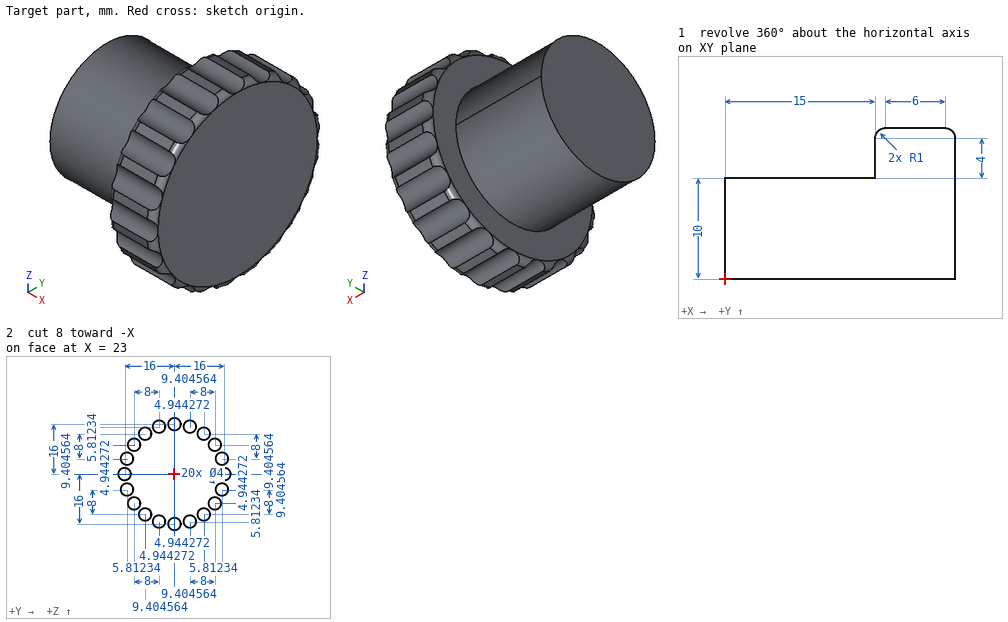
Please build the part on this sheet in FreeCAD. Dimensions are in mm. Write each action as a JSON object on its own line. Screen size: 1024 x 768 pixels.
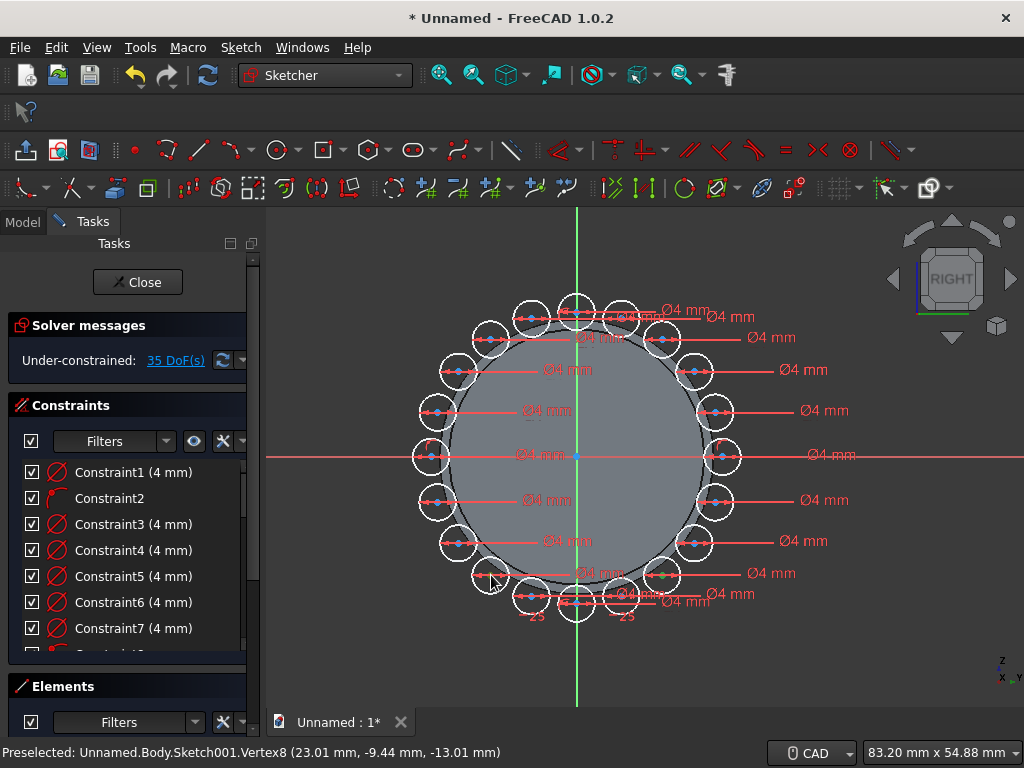
{"action": "left_click", "coordinate": [668, 150]}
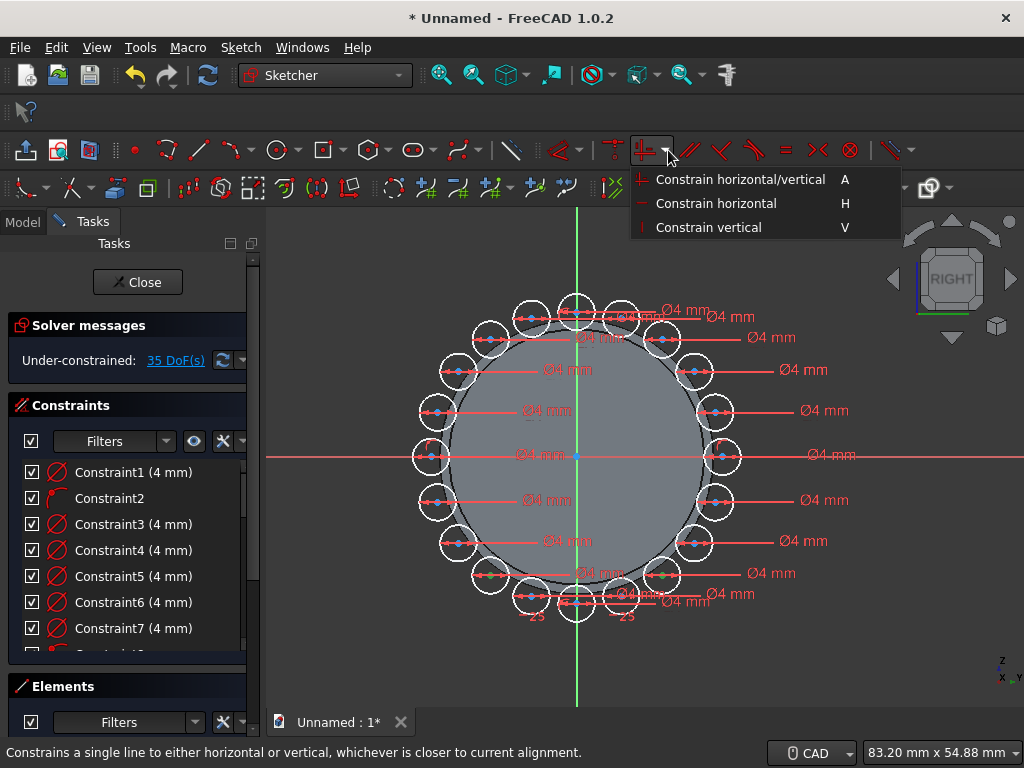
{"action": "left_click", "coordinate": [766, 203]}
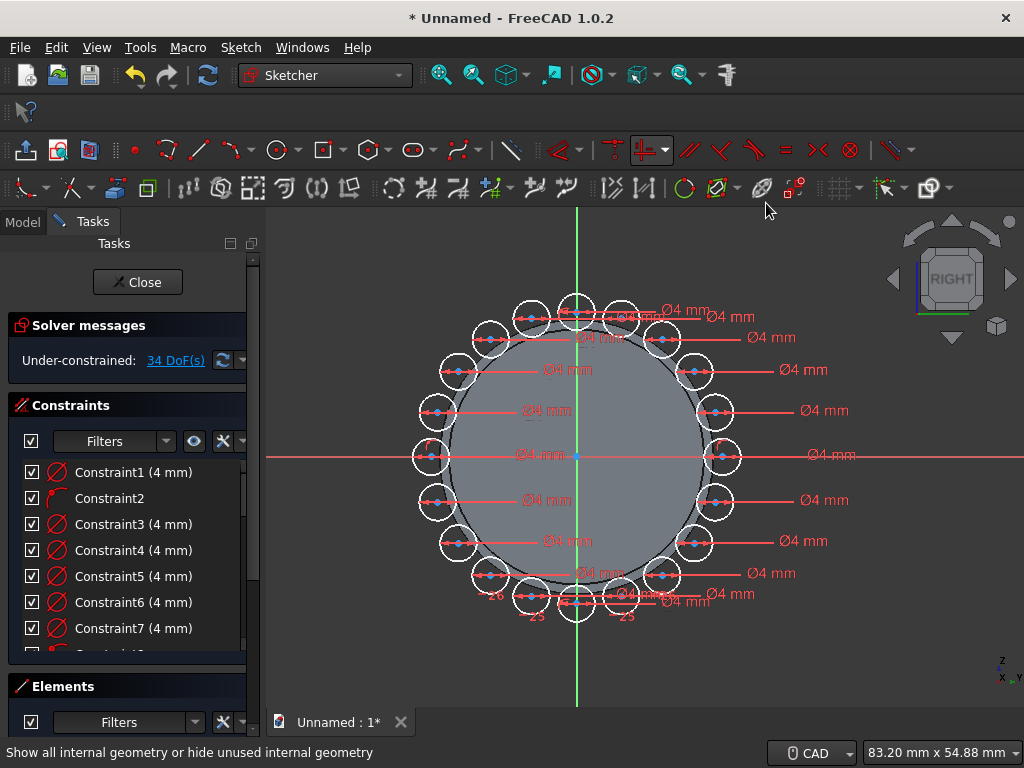
{"action": "left_click", "coordinate": [694, 543]}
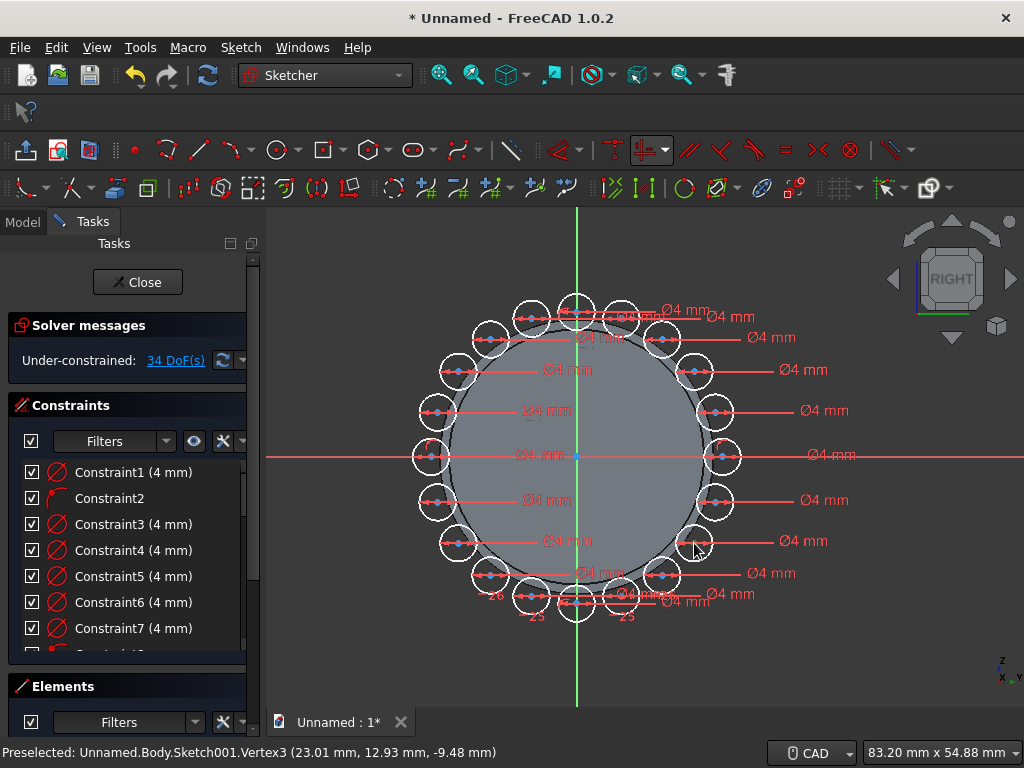
{"action": "left_click", "coordinate": [458, 543]}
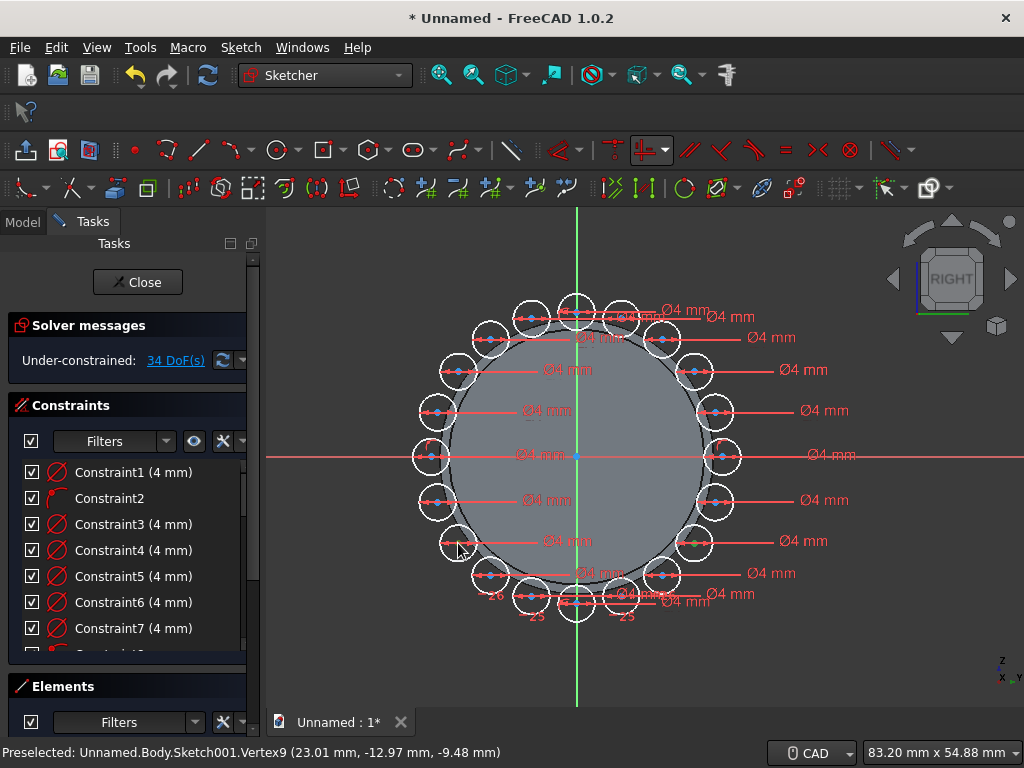
{"action": "left_click", "coordinate": [668, 150]}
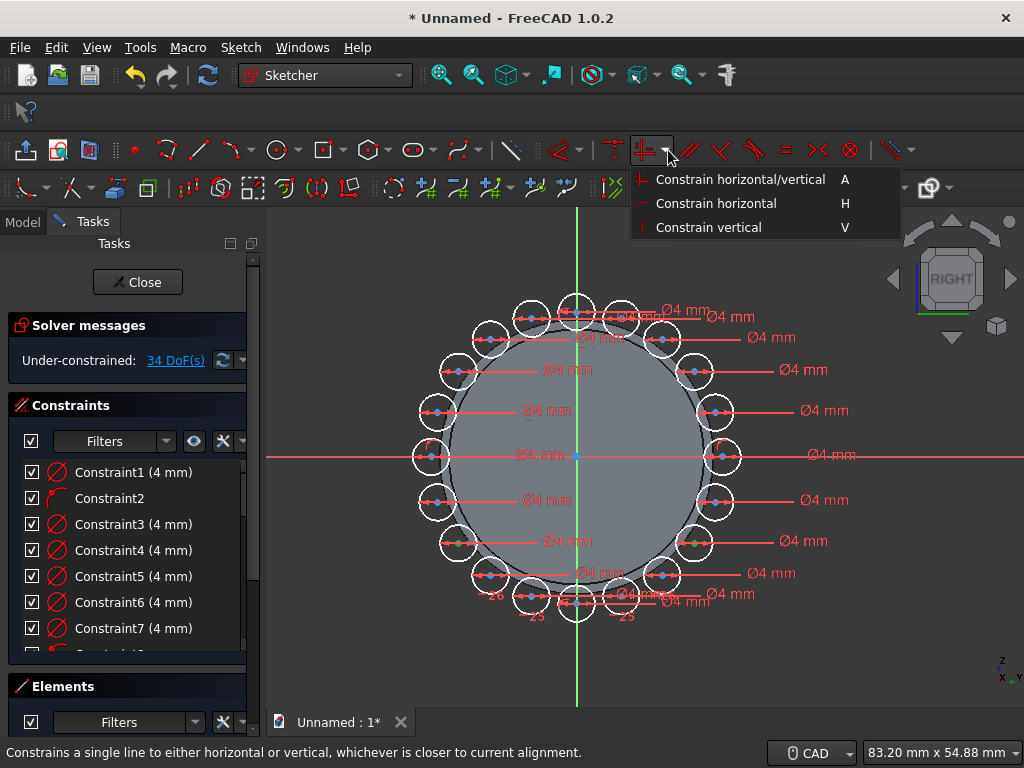
{"action": "left_click", "coordinate": [766, 203]}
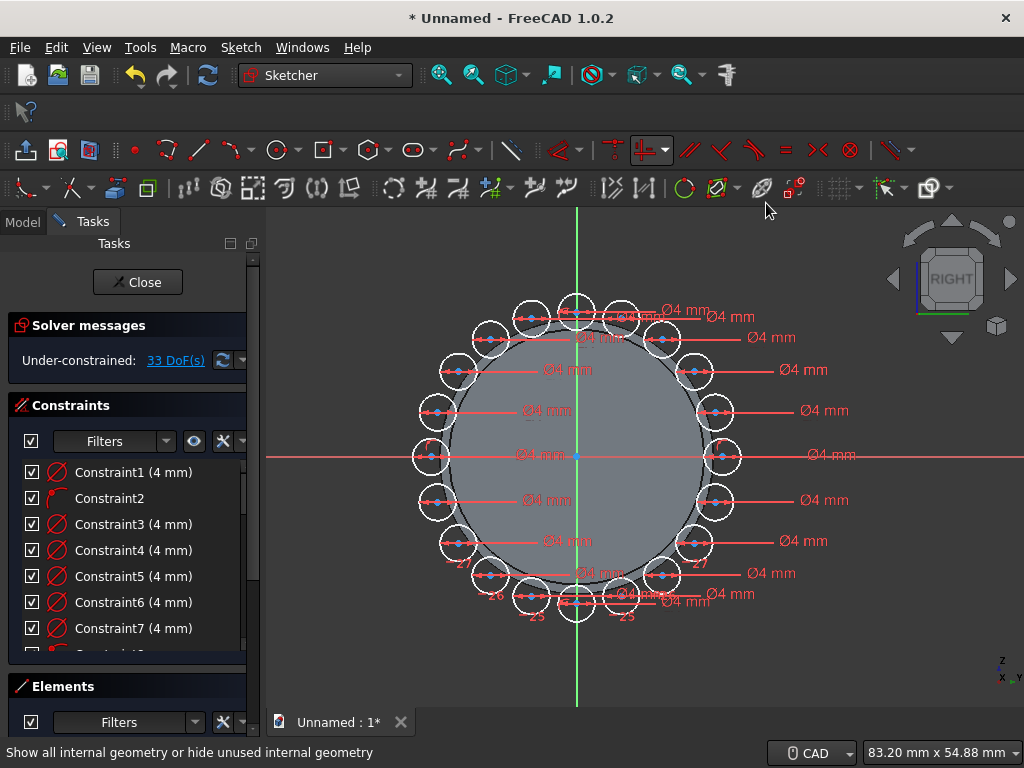
{"action": "left_click", "coordinate": [438, 502]}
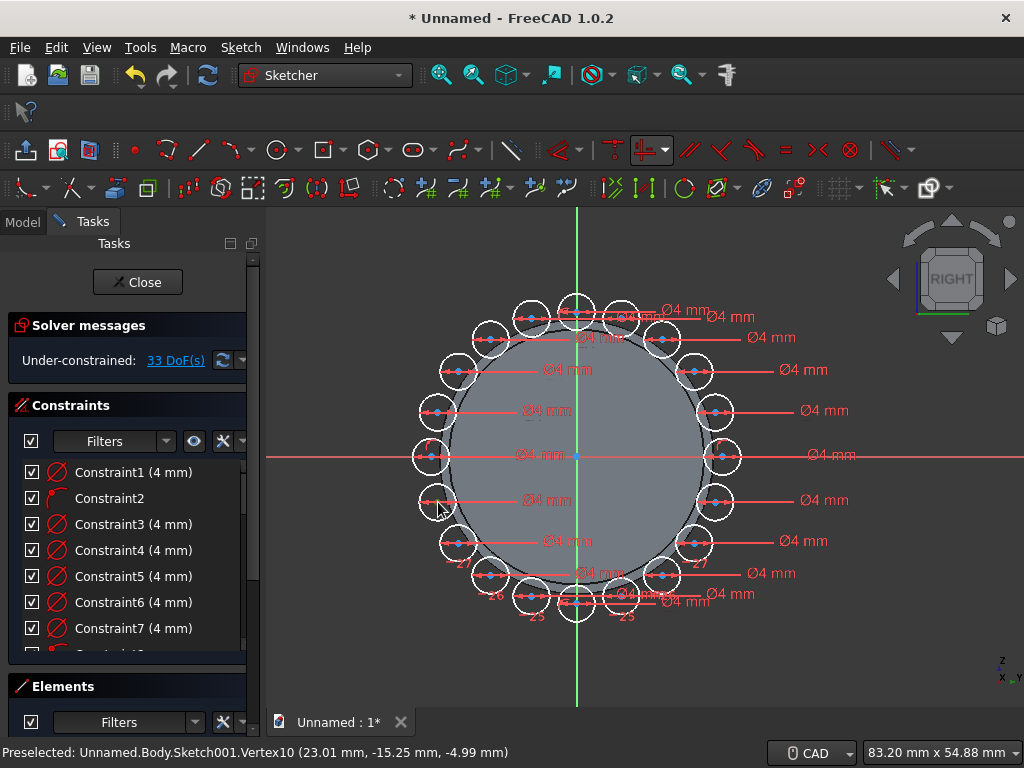
{"action": "left_click", "coordinate": [438, 413]}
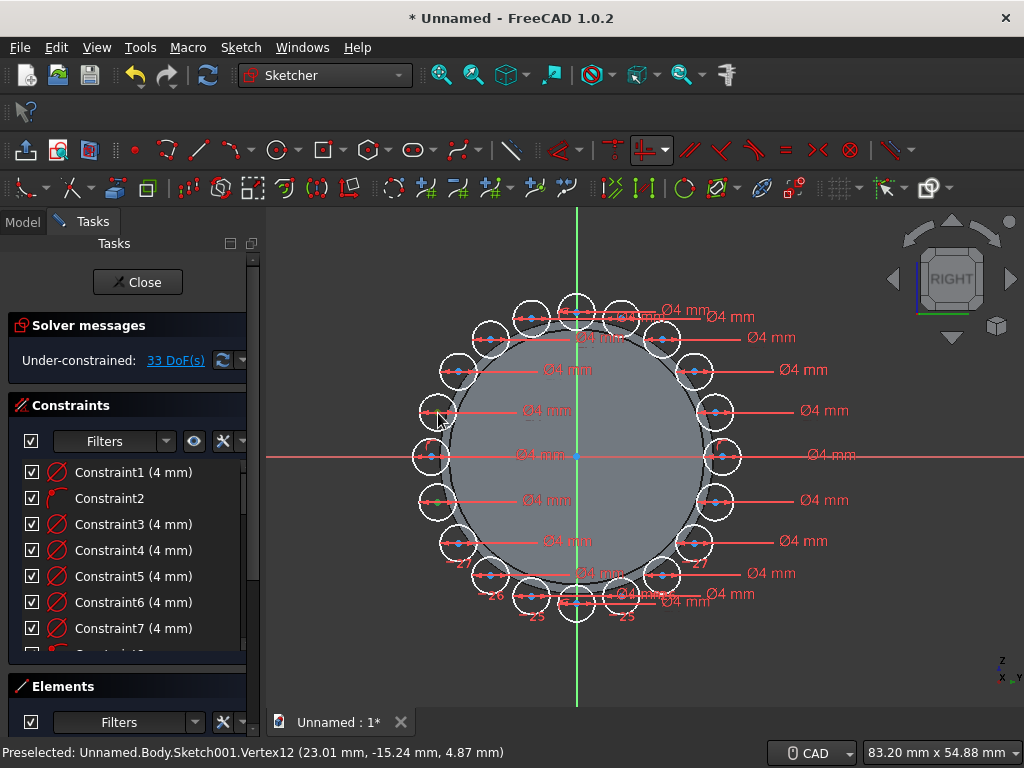
{"action": "key", "text": "v"}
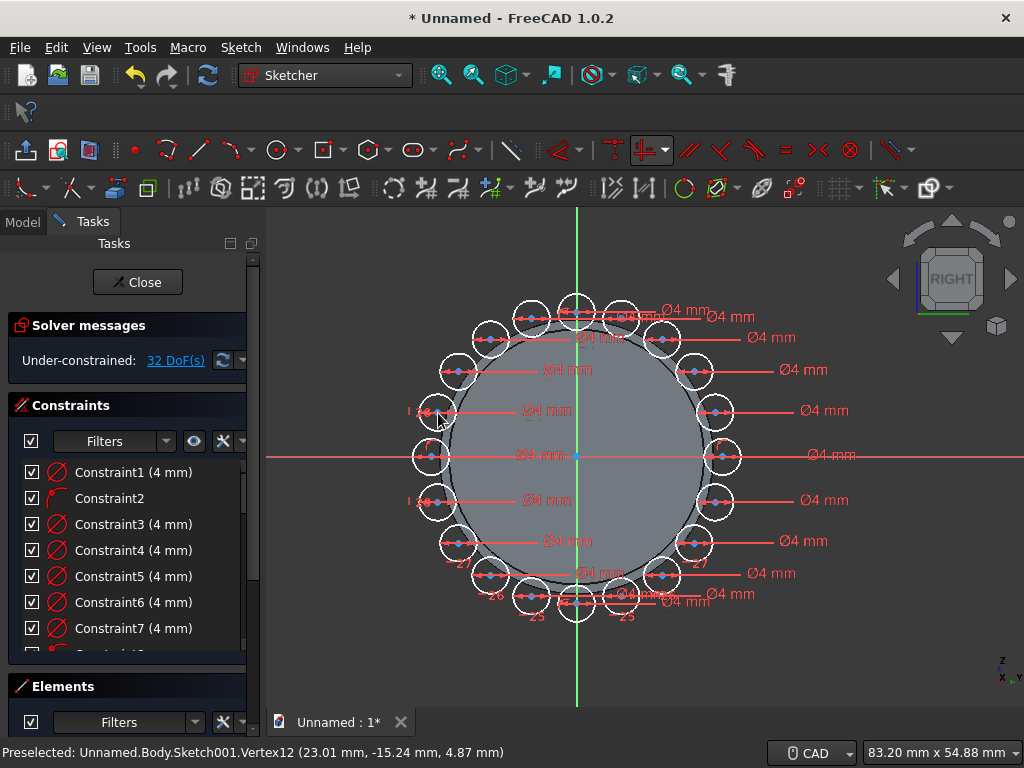
{"action": "left_click", "coordinate": [458, 543]}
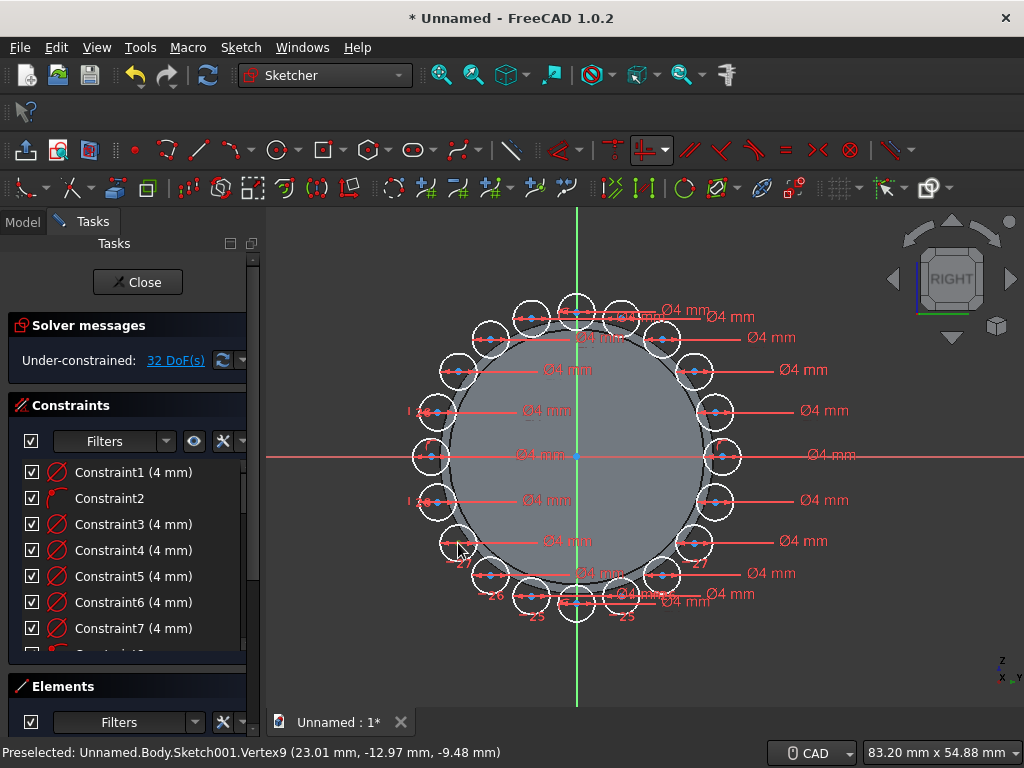
{"action": "left_click", "coordinate": [459, 372]}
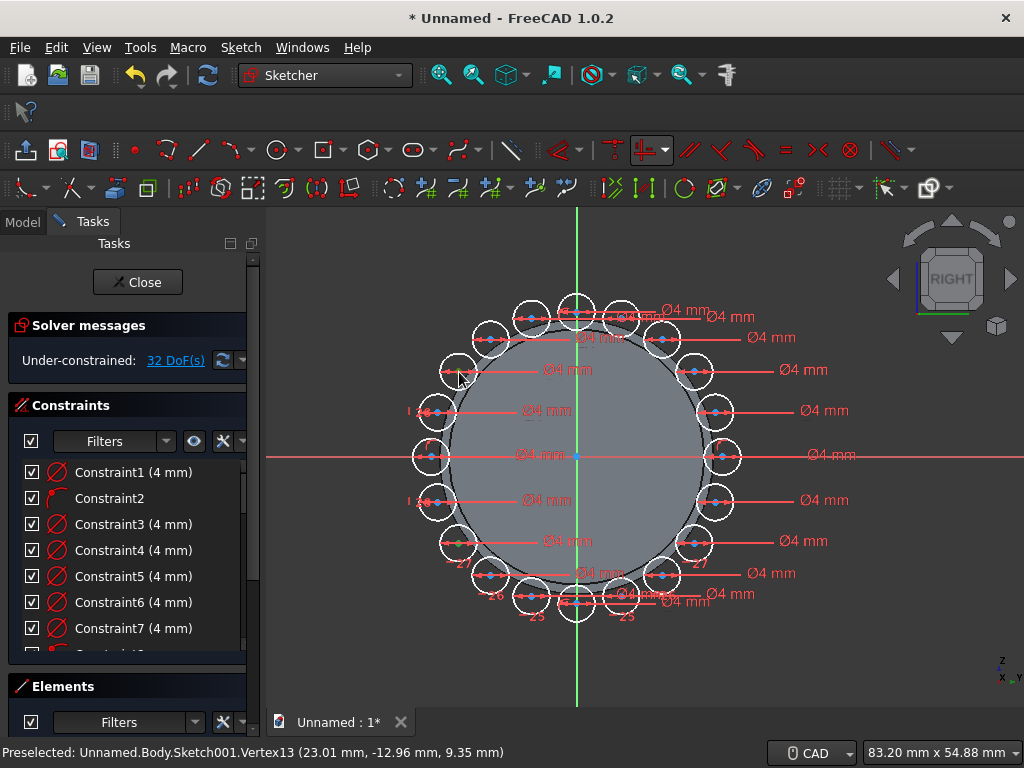
{"action": "left_click", "coordinate": [668, 150]}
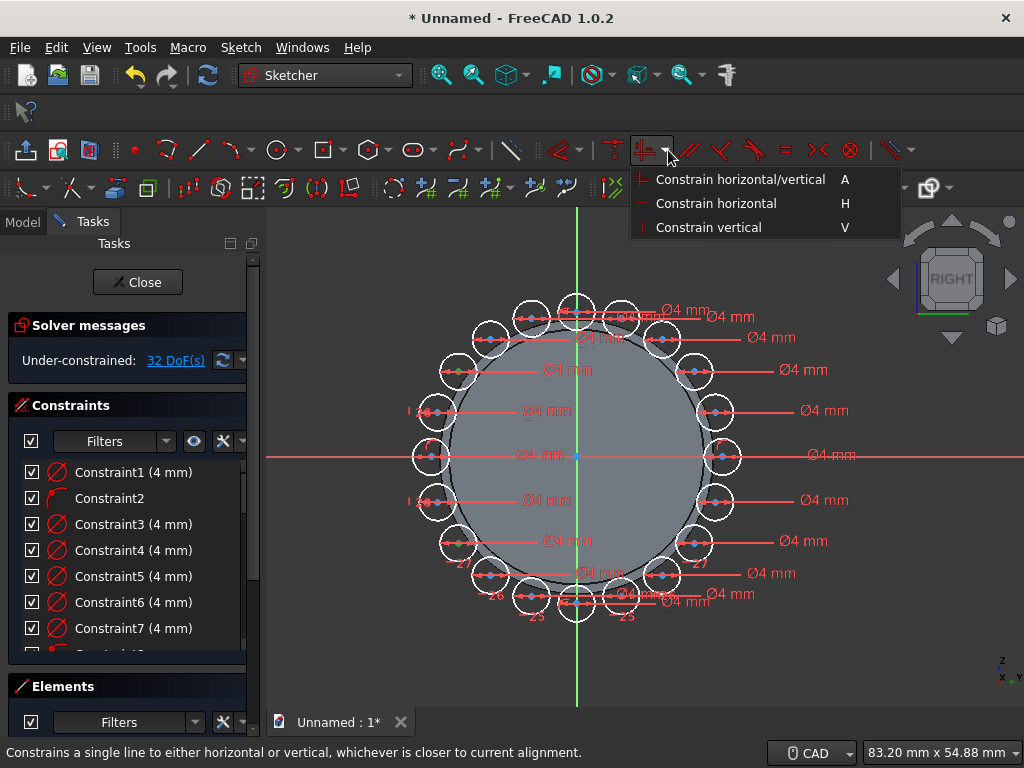
{"action": "left_click", "coordinate": [766, 227]}